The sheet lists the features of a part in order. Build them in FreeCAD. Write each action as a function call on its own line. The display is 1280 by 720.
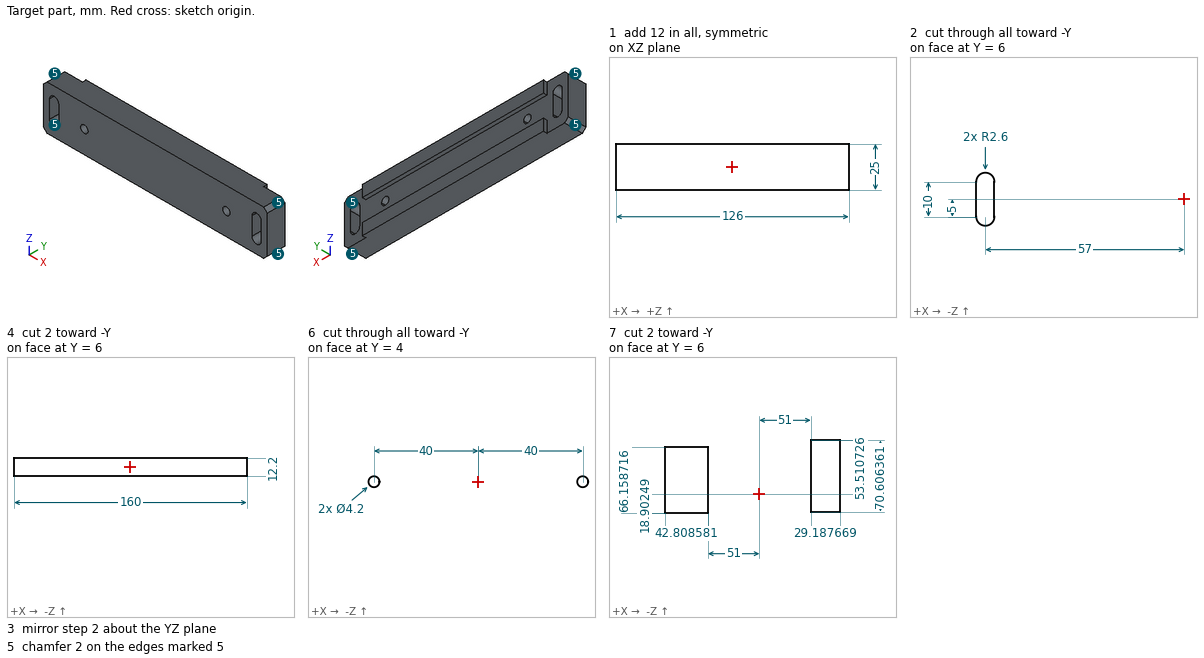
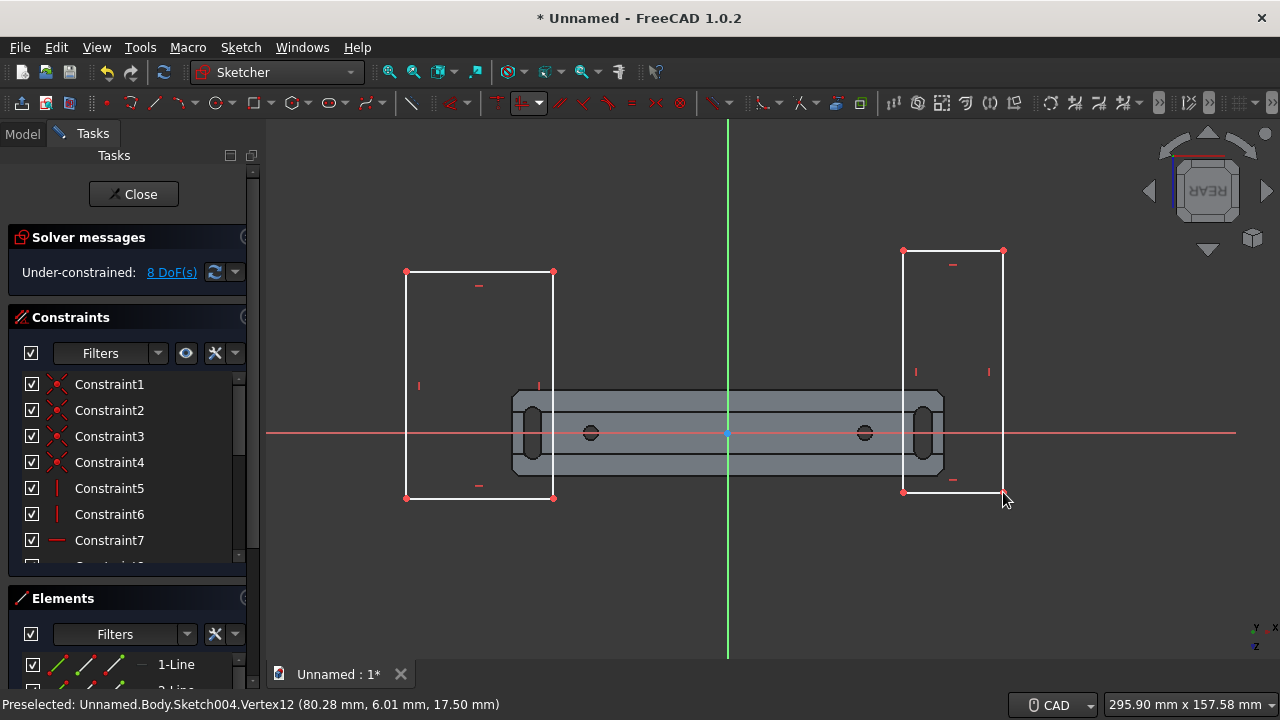
click(450, 104)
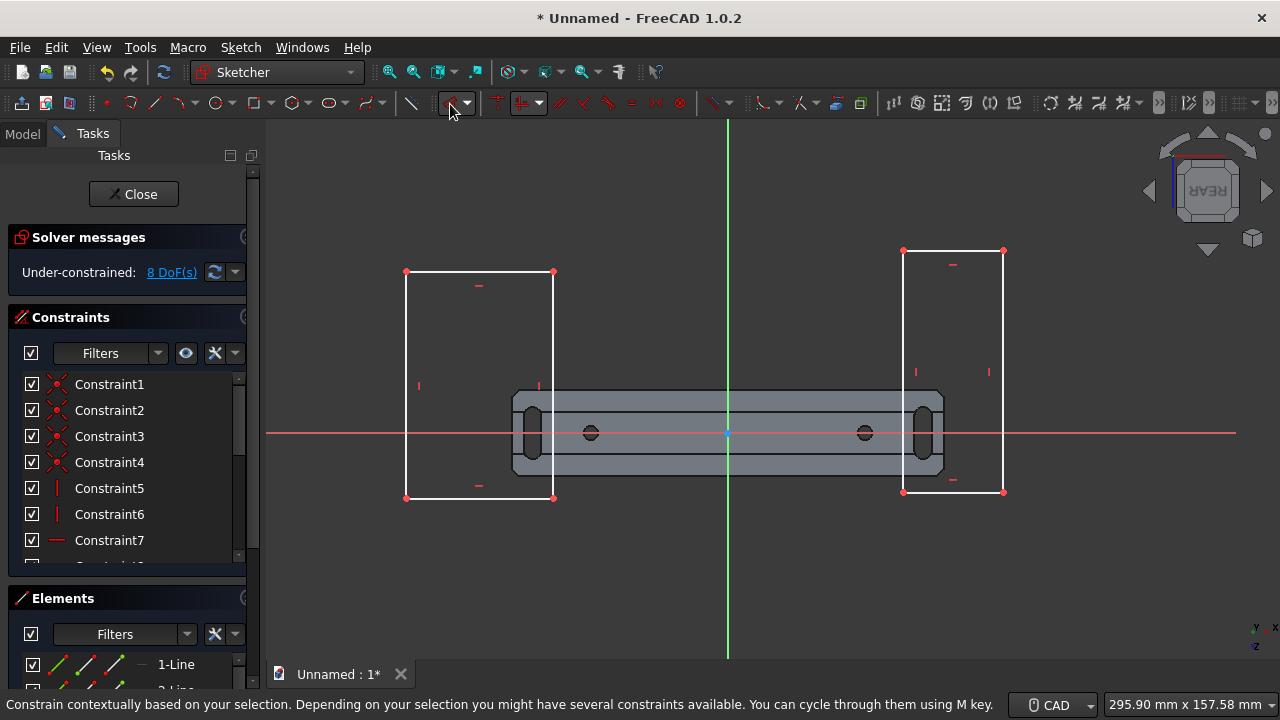
click(553, 499)
click(640, 533)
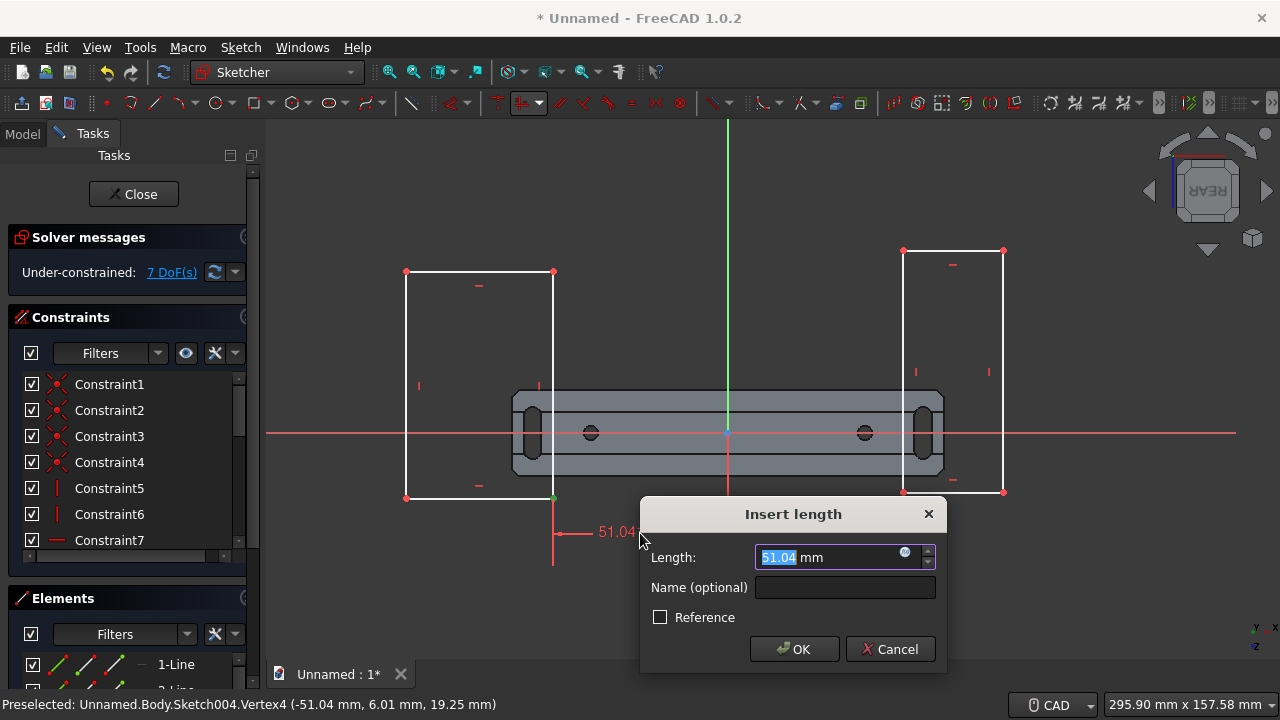
text(51)
key(Return)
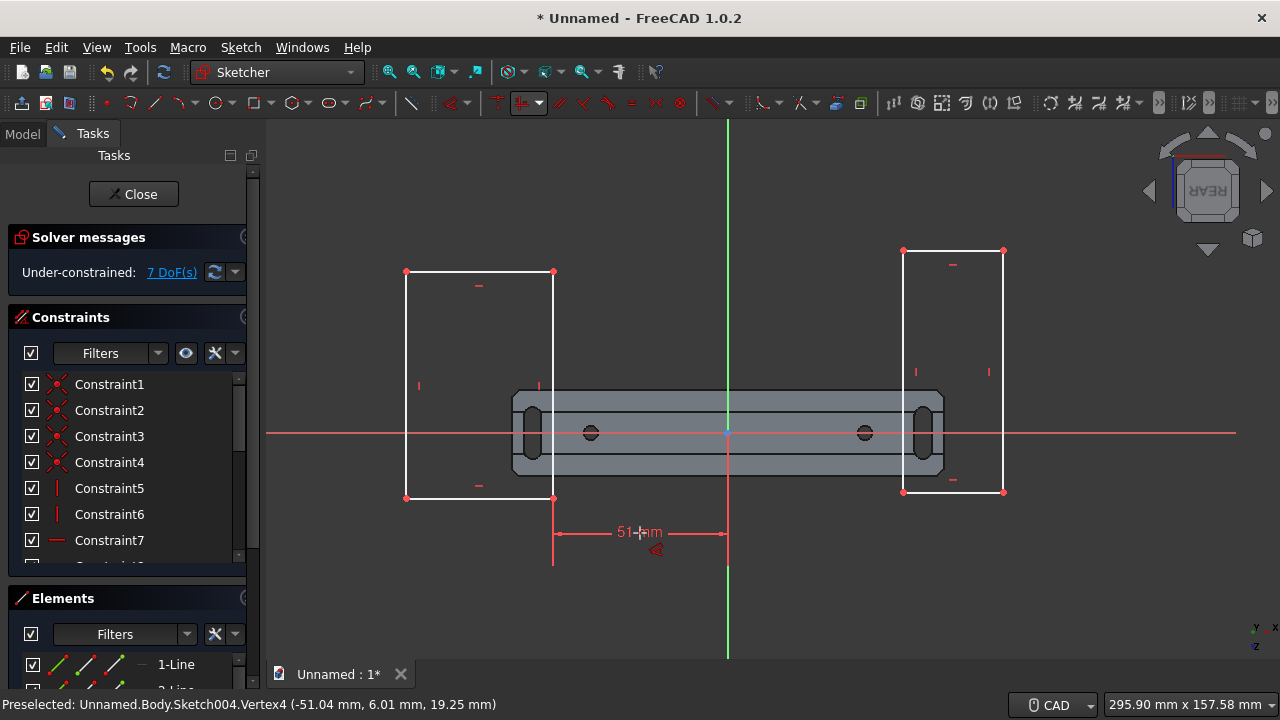
click(903, 251)
click(815, 217)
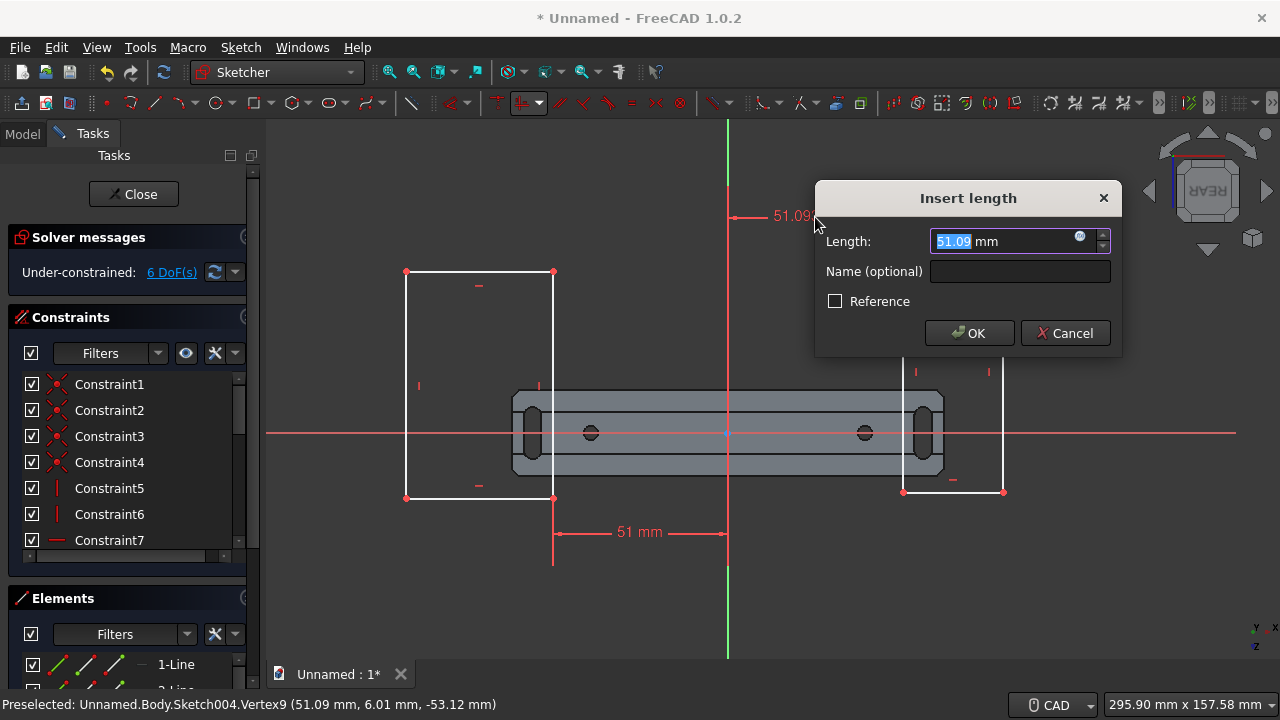
text(51)
key(Return)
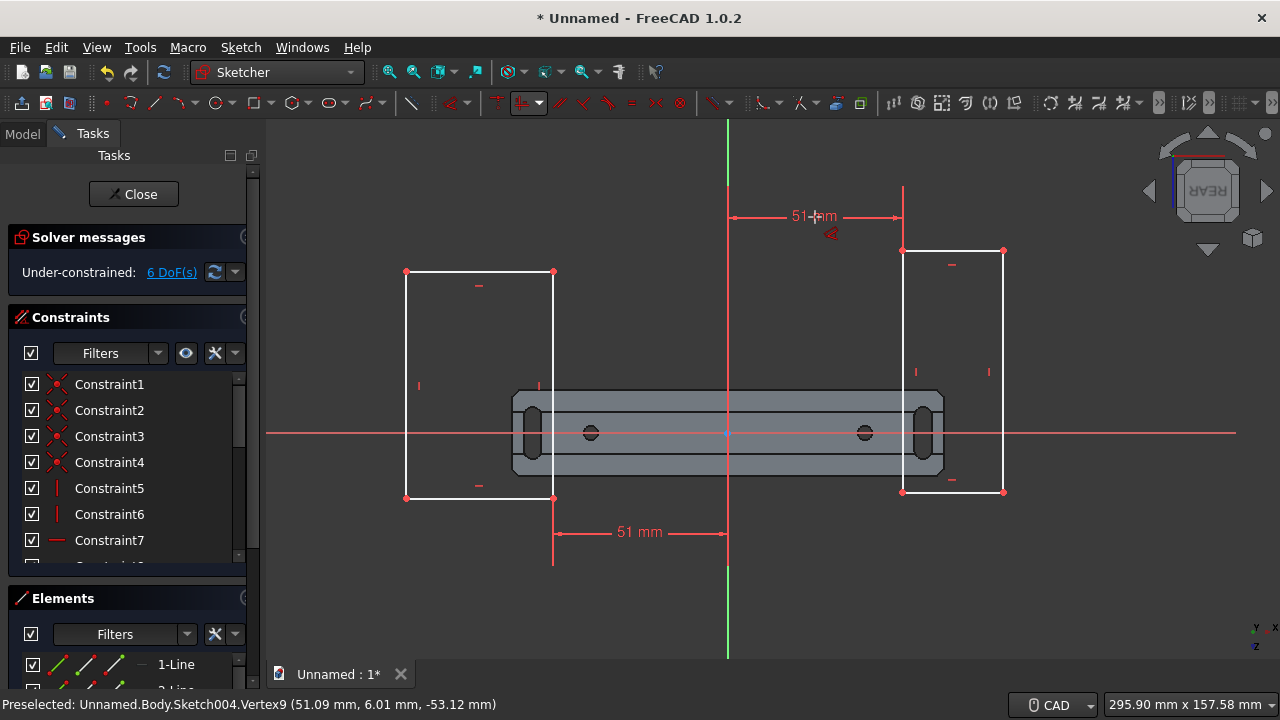
click(406, 340)
click(372, 386)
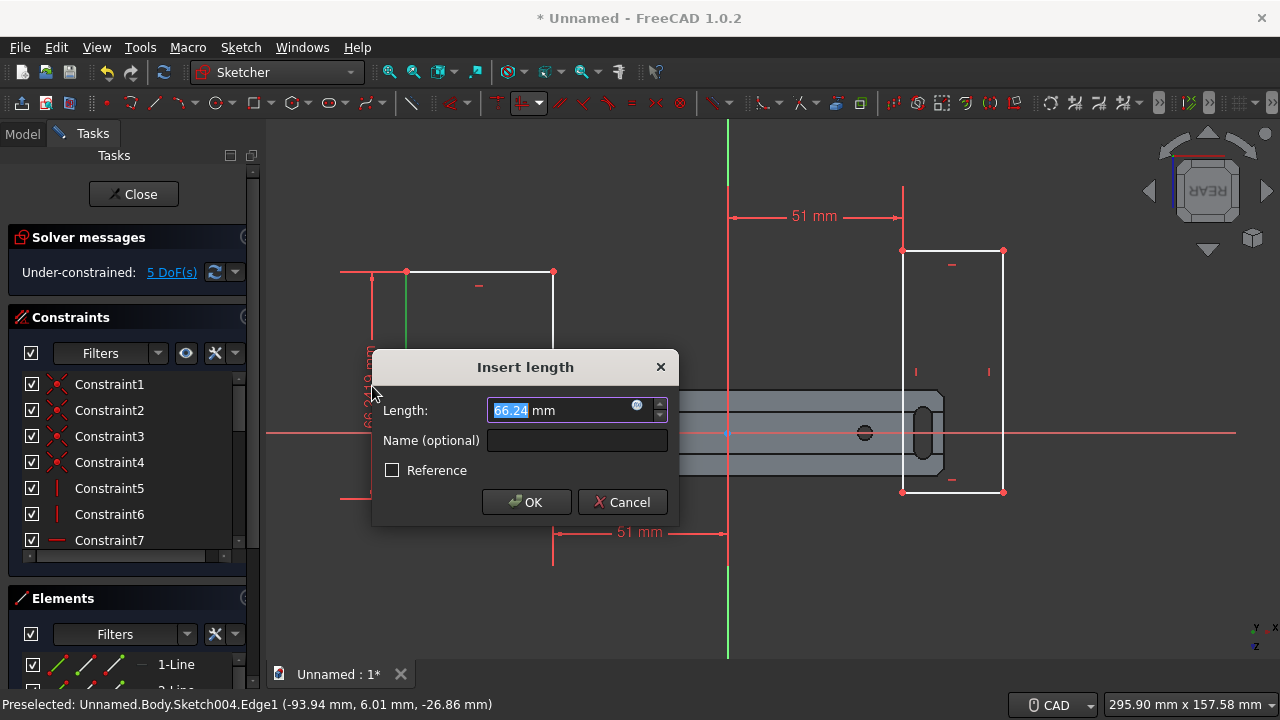
text(66.158716)
key(Return)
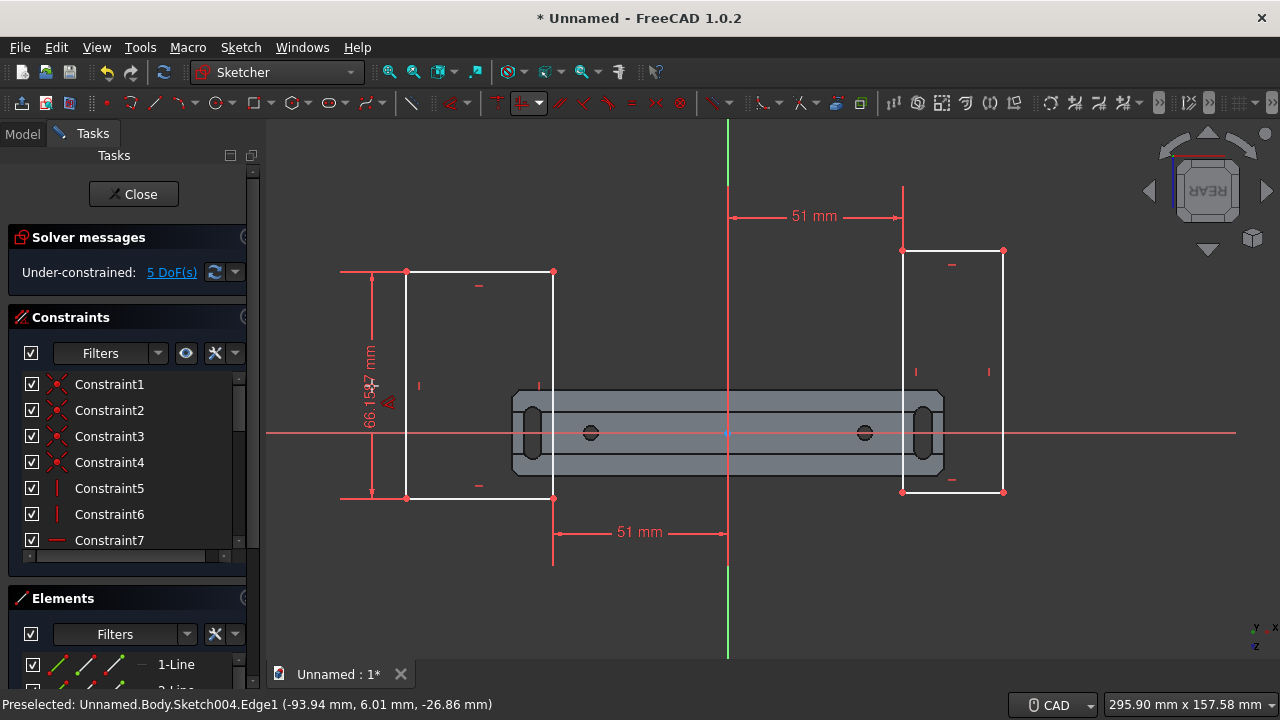
click(450, 499)
click(480, 533)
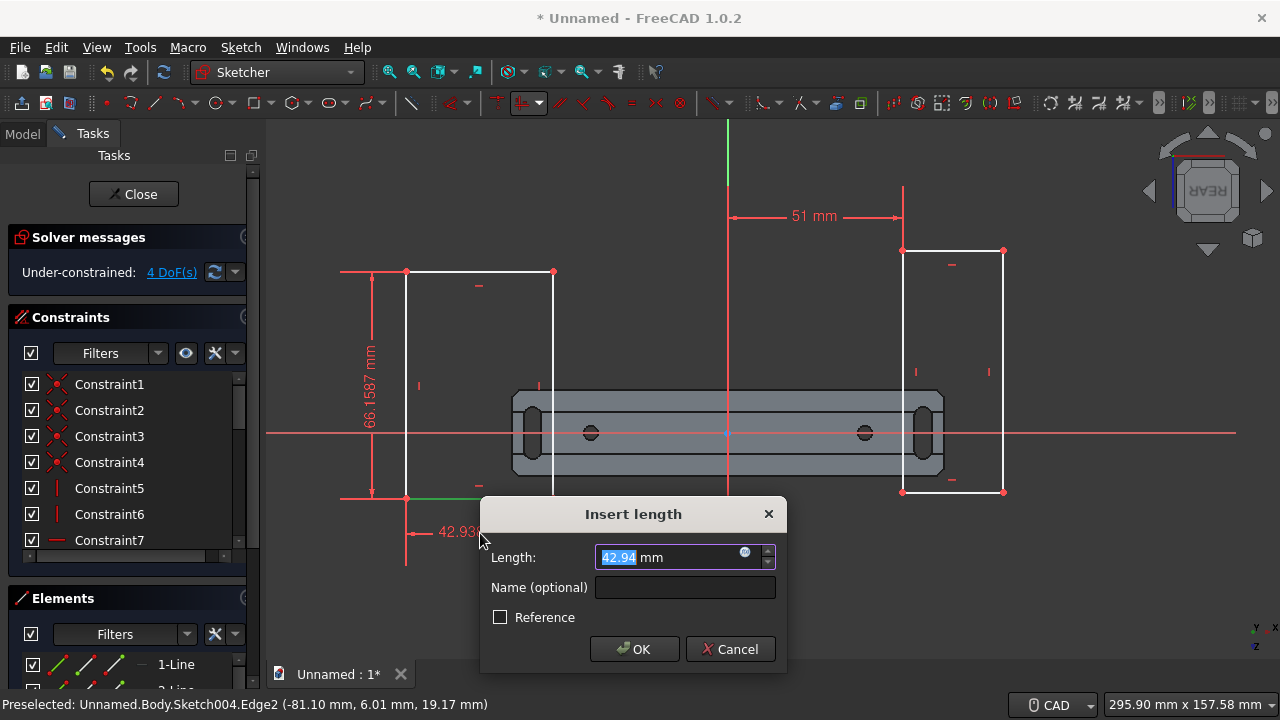
text(42.808581)
key(Return)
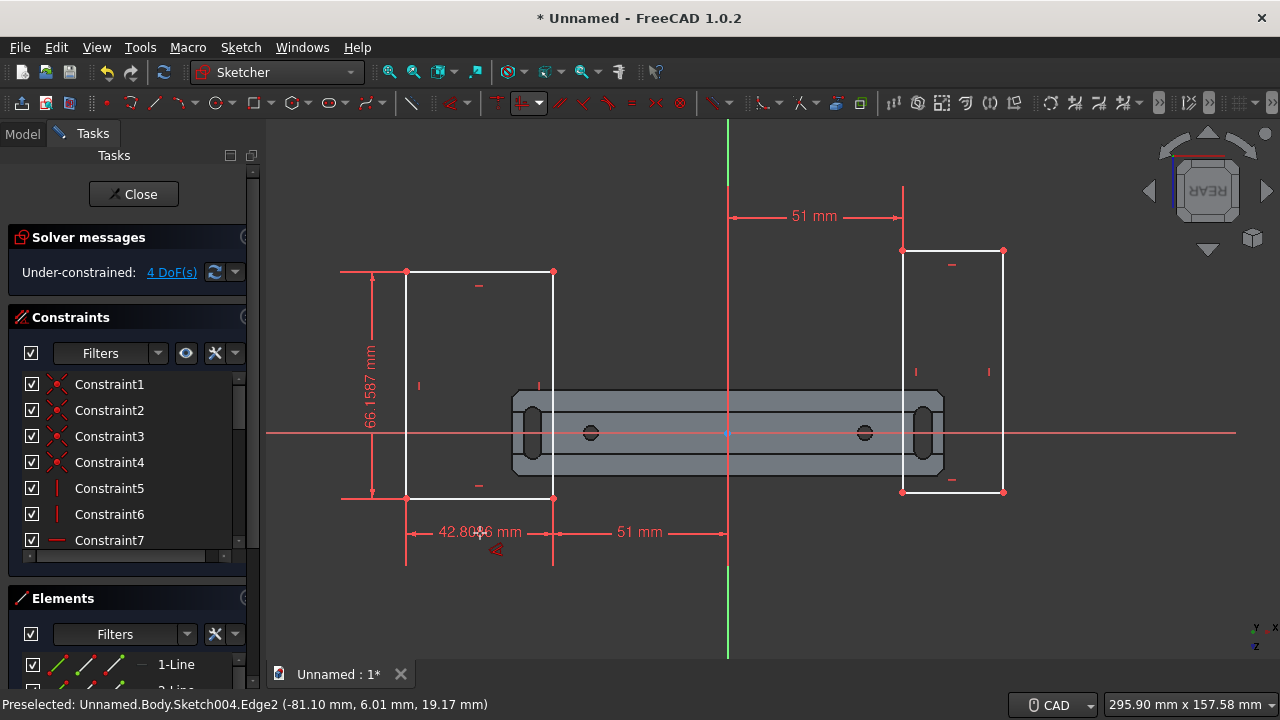
click(903, 324)
click(937, 372)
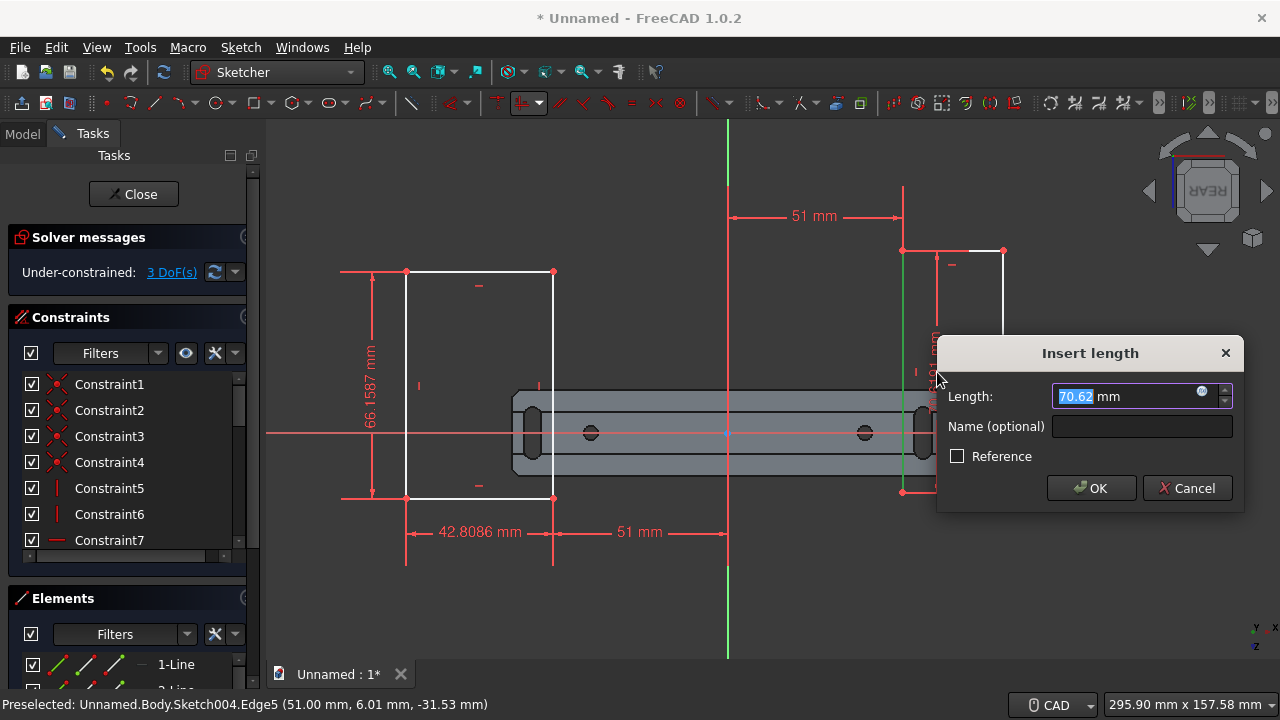
text(70.606361)
key(Return)